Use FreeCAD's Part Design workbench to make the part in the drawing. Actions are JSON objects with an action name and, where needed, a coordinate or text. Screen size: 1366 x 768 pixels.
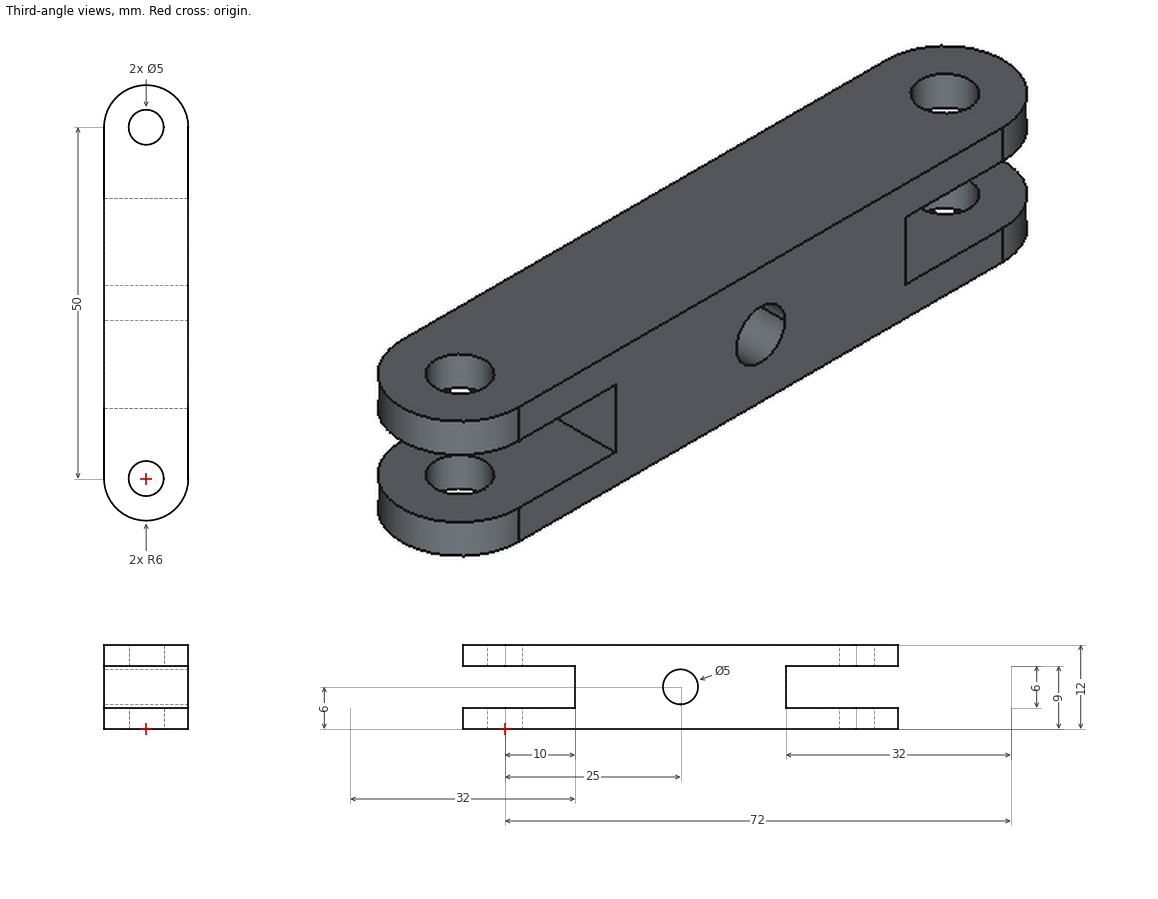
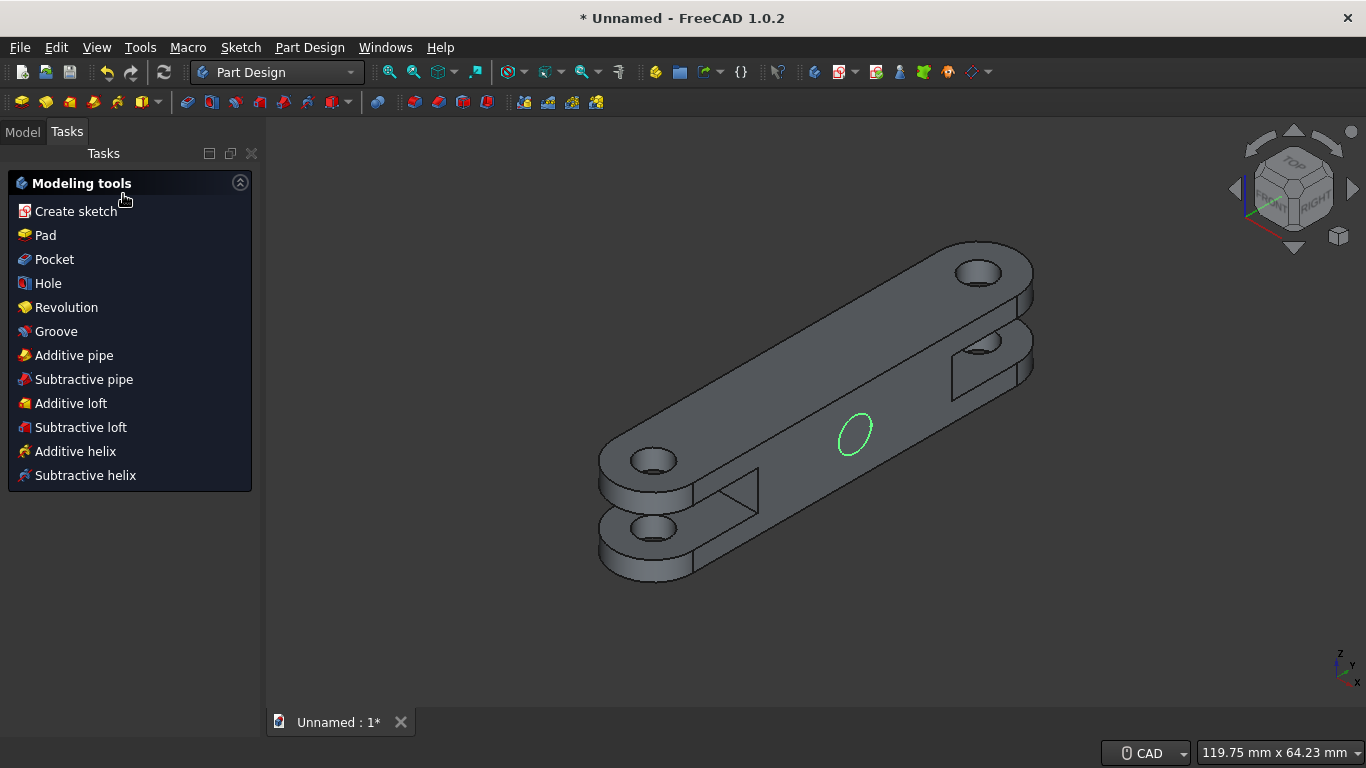
{"action": "left_click", "coordinate": [188, 102]}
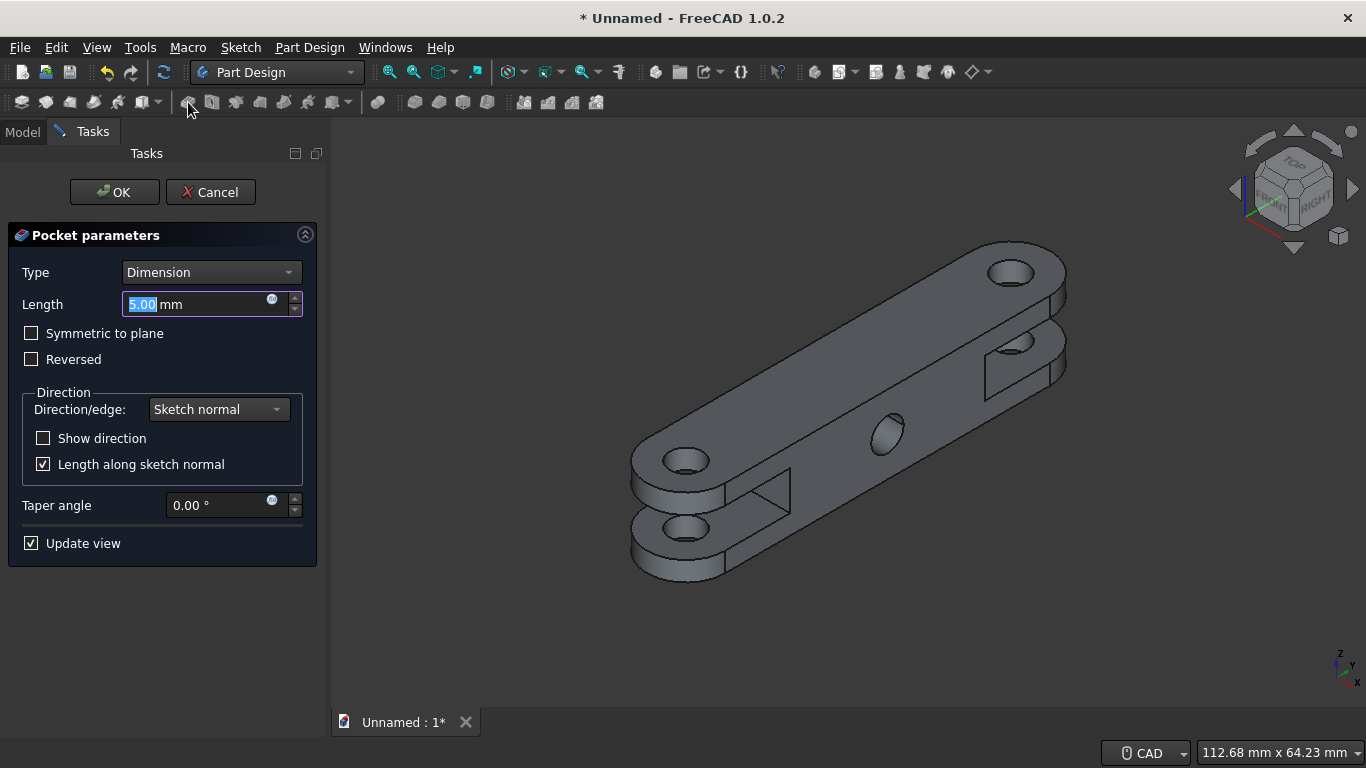
{"action": "left_click", "coordinate": [212, 272]}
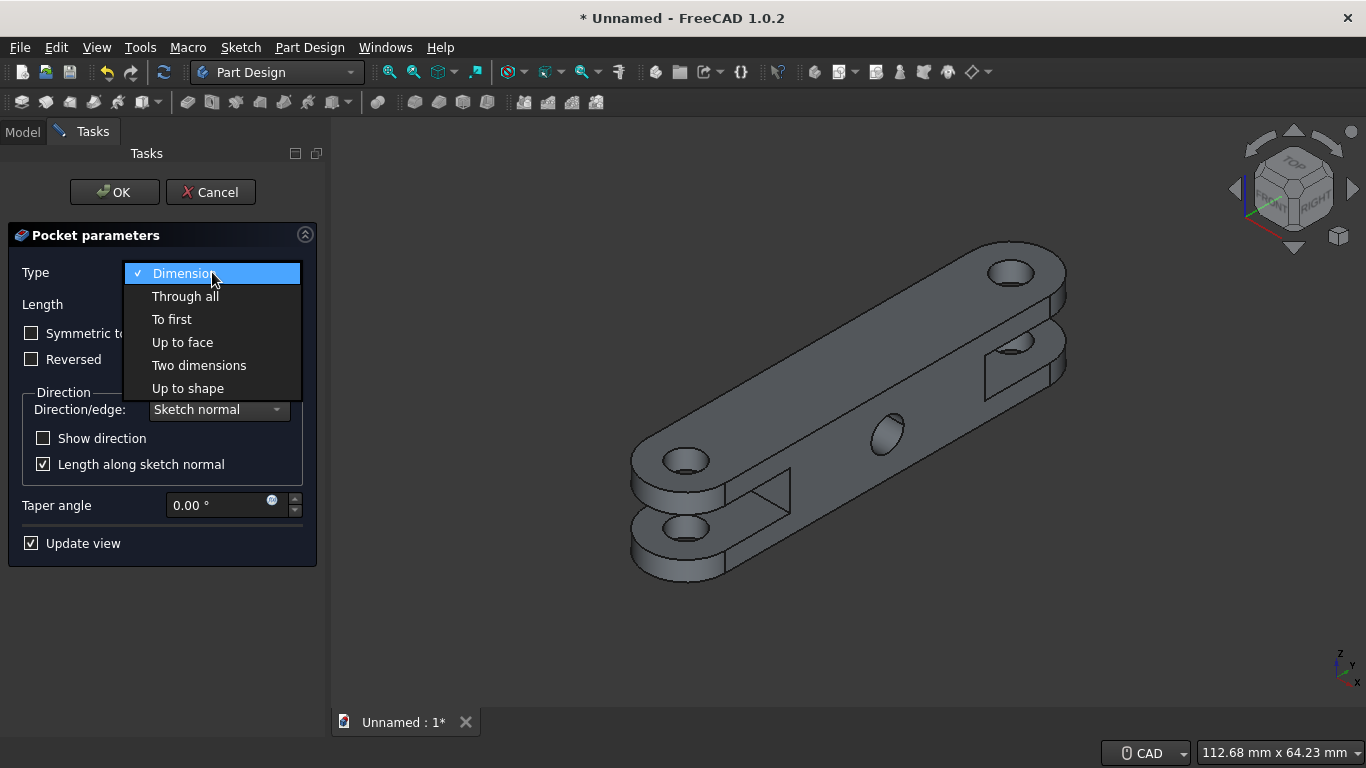
{"action": "left_click", "coordinate": [212, 296]}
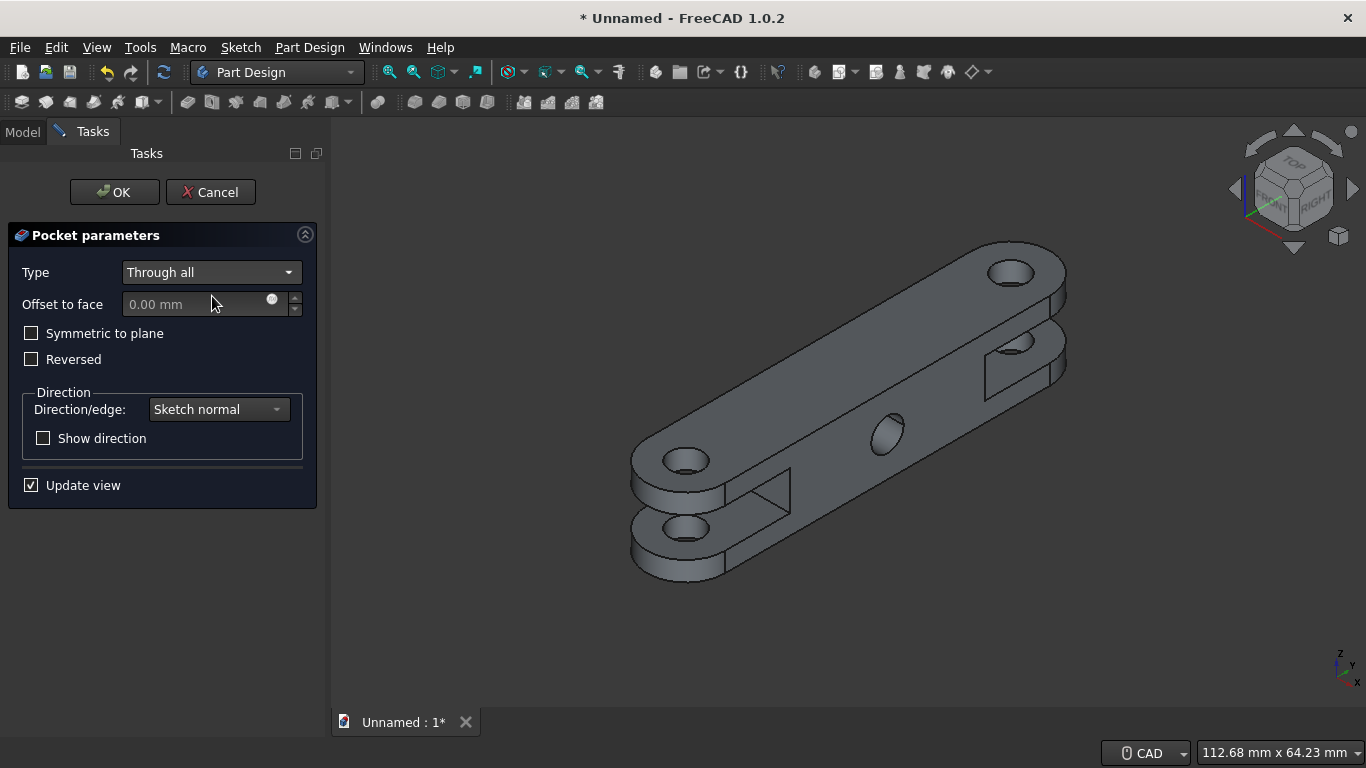
{"action": "left_click", "coordinate": [115, 192]}